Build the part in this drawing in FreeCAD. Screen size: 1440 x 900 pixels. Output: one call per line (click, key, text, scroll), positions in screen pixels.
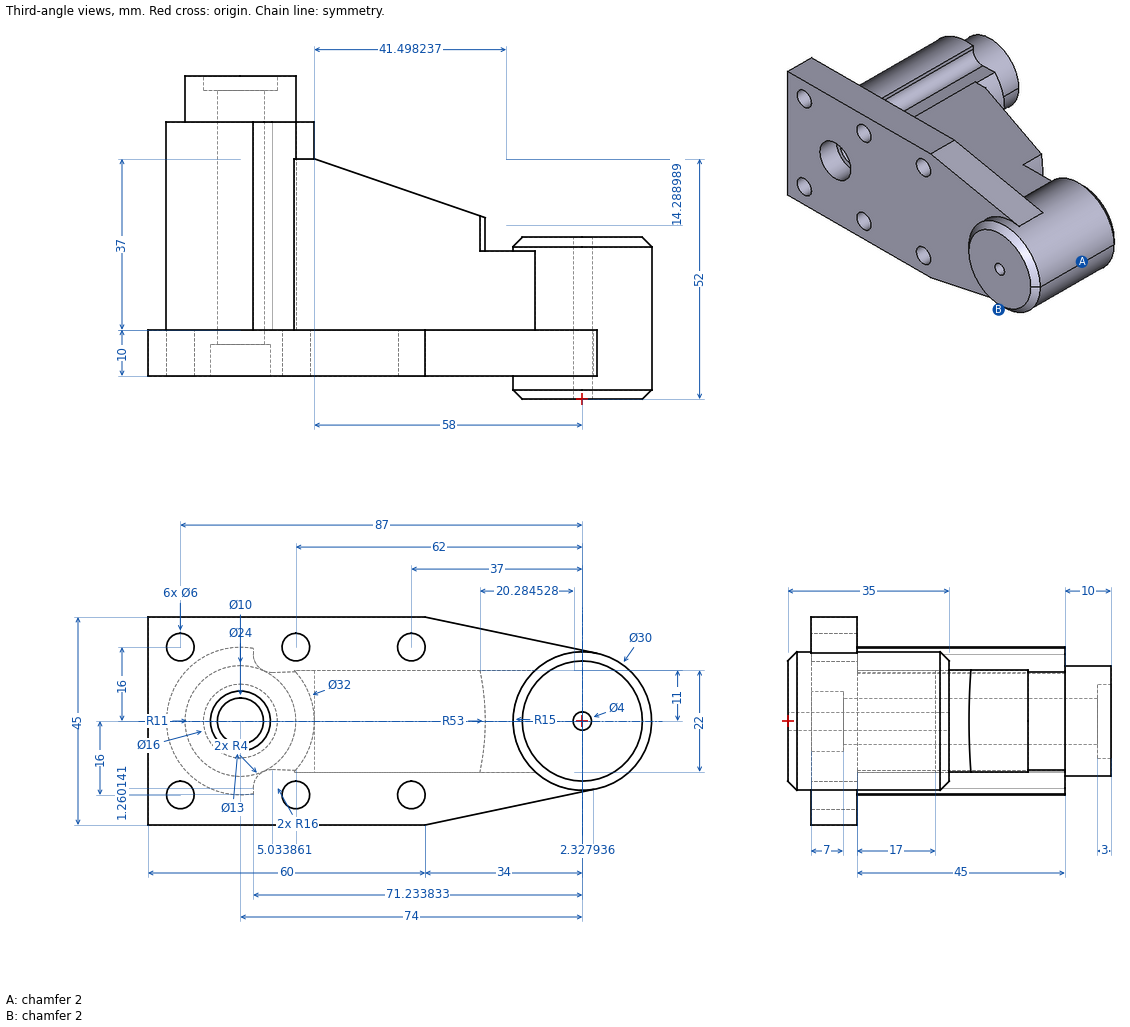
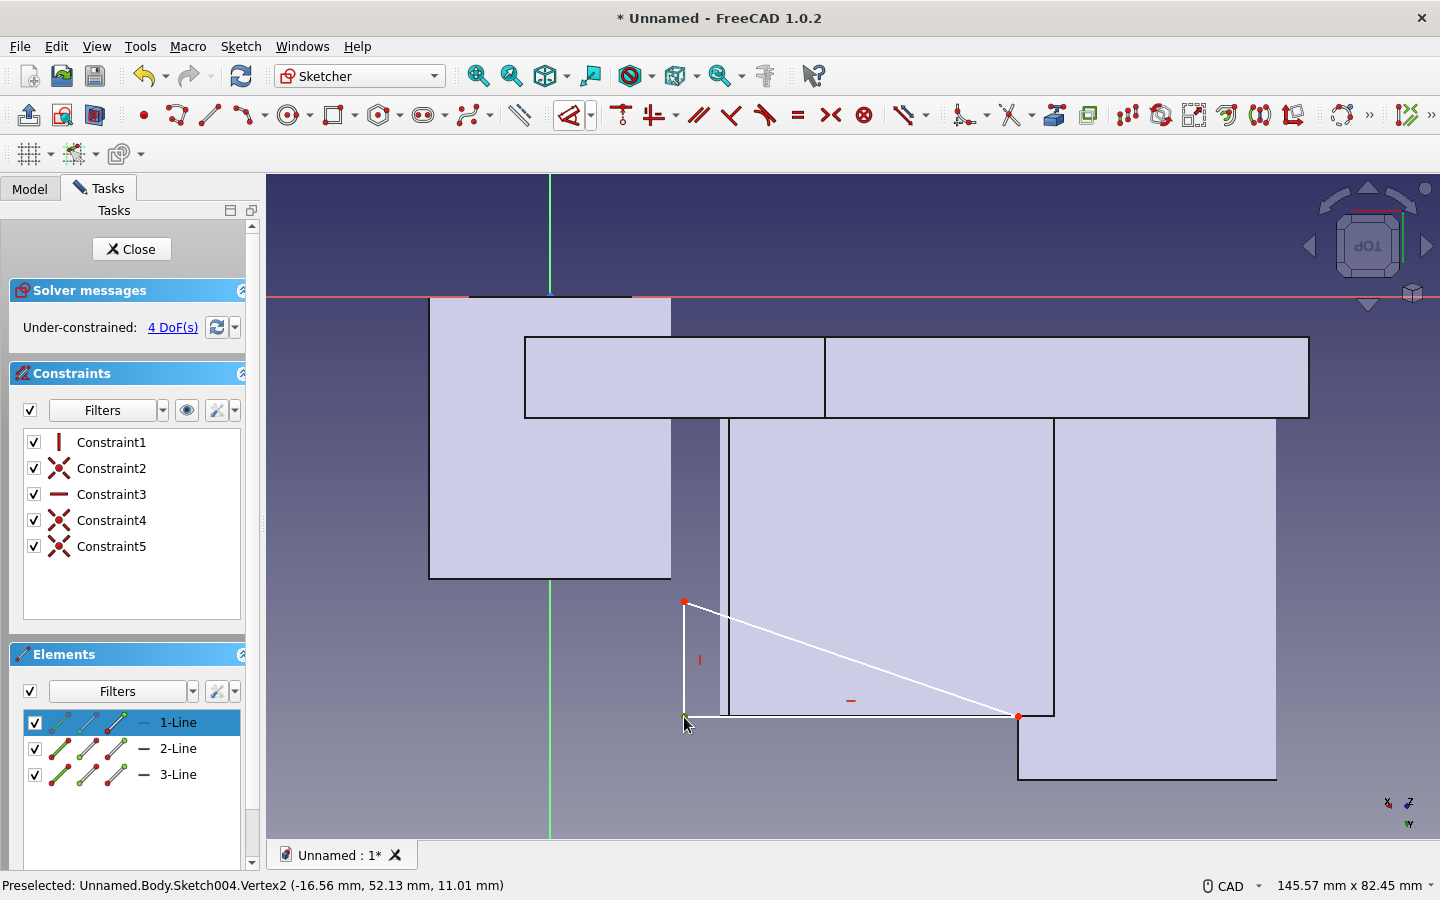
click(590, 116)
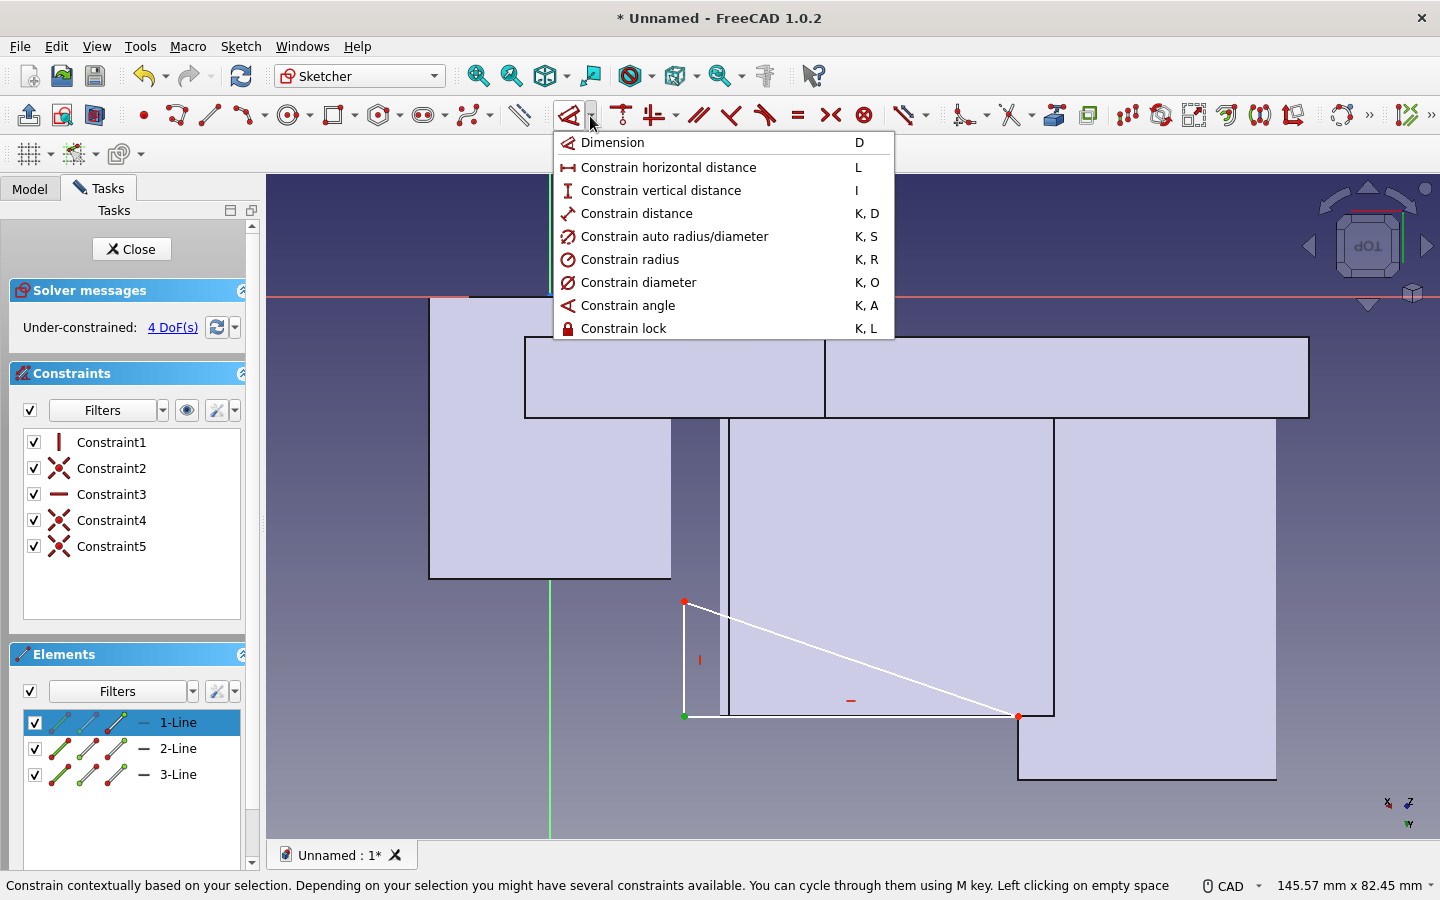
click(724, 190)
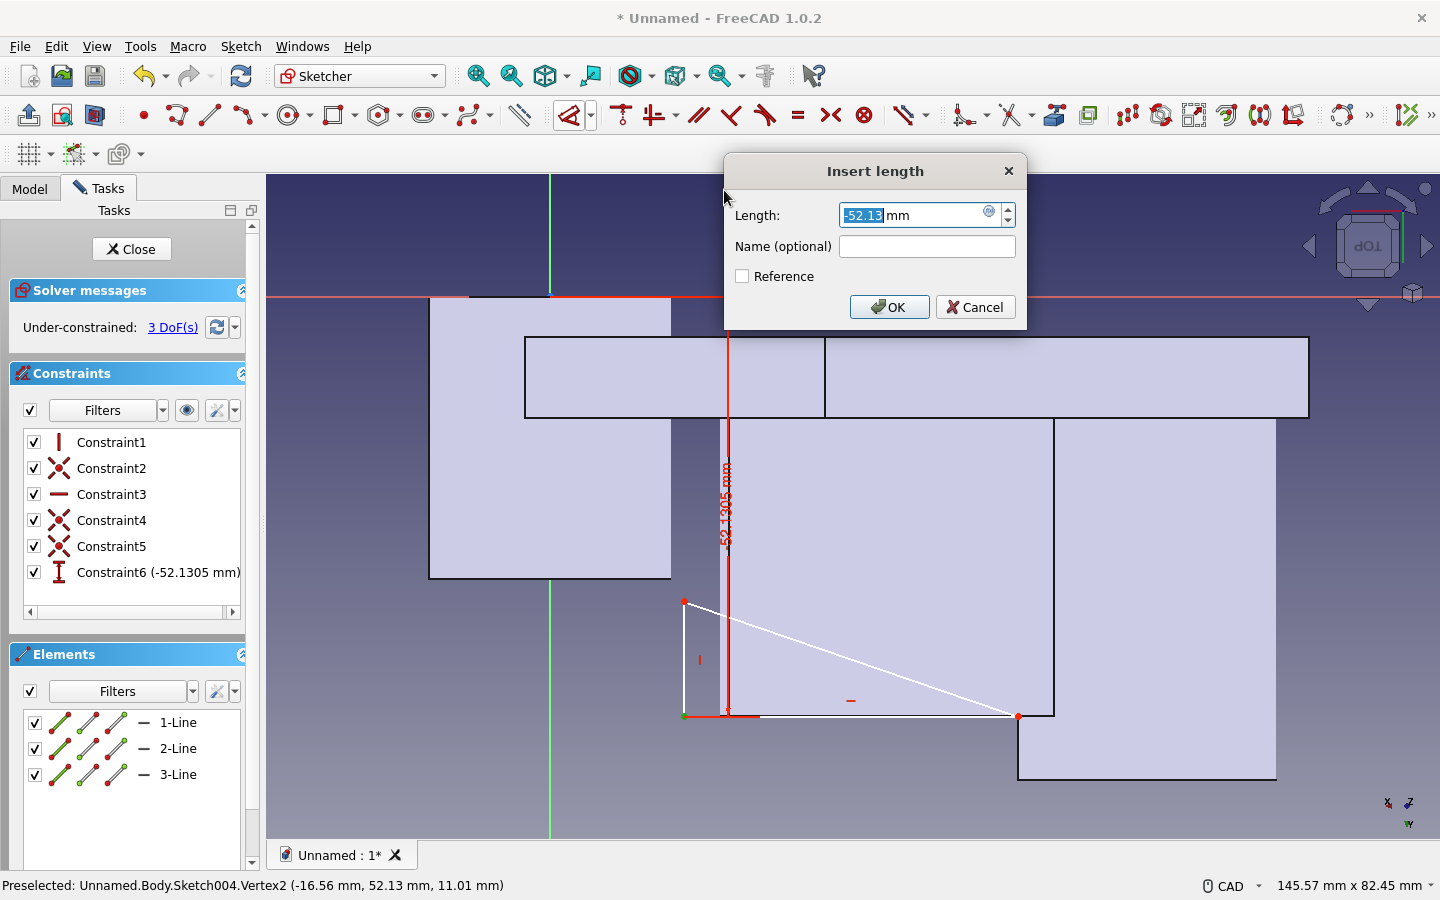
text(-52)
key(Return)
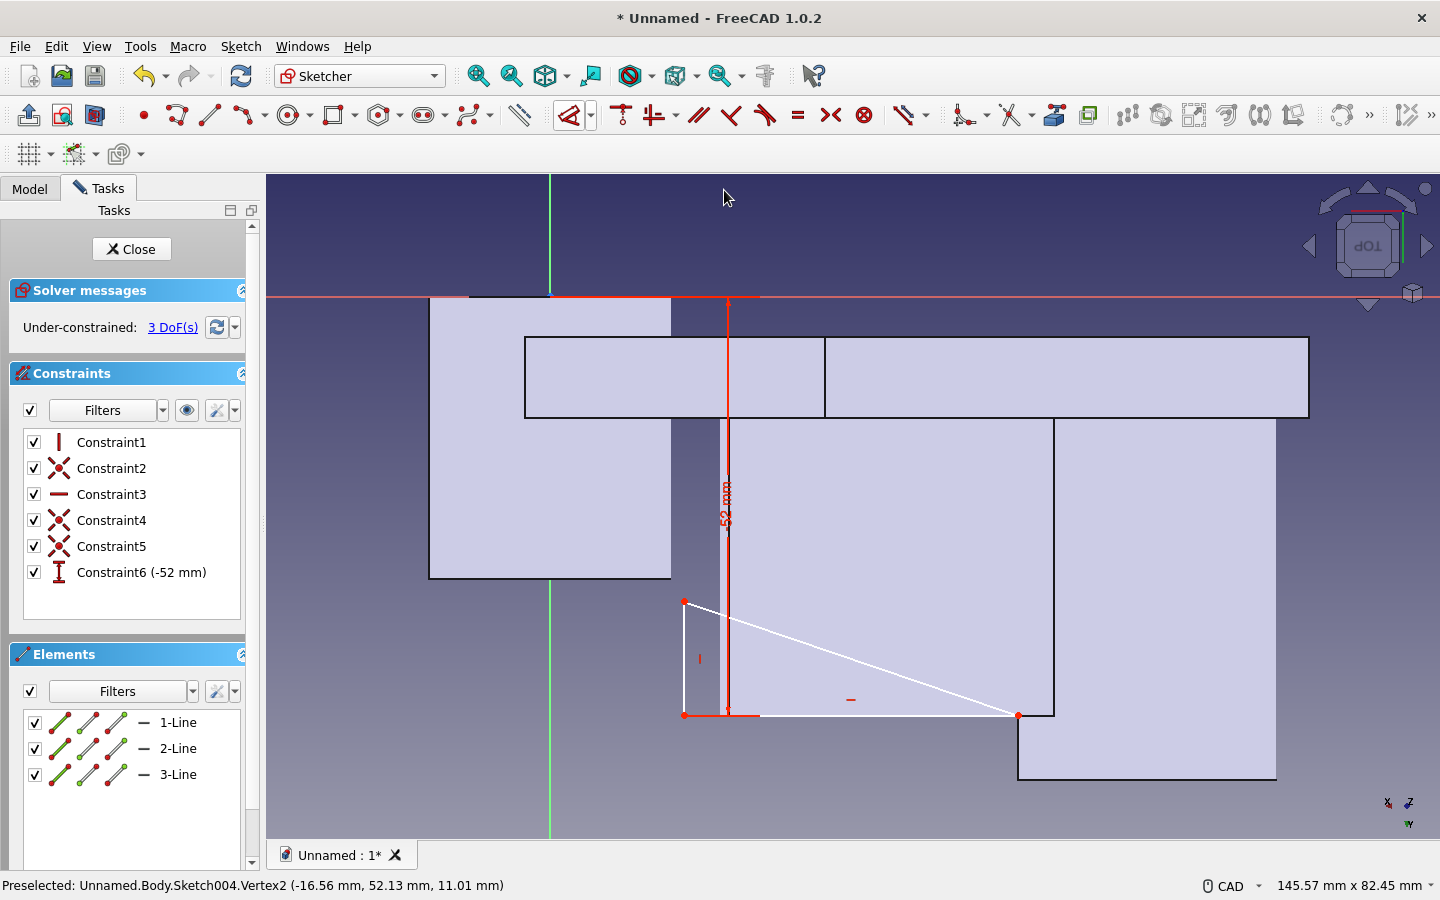
click(1018, 716)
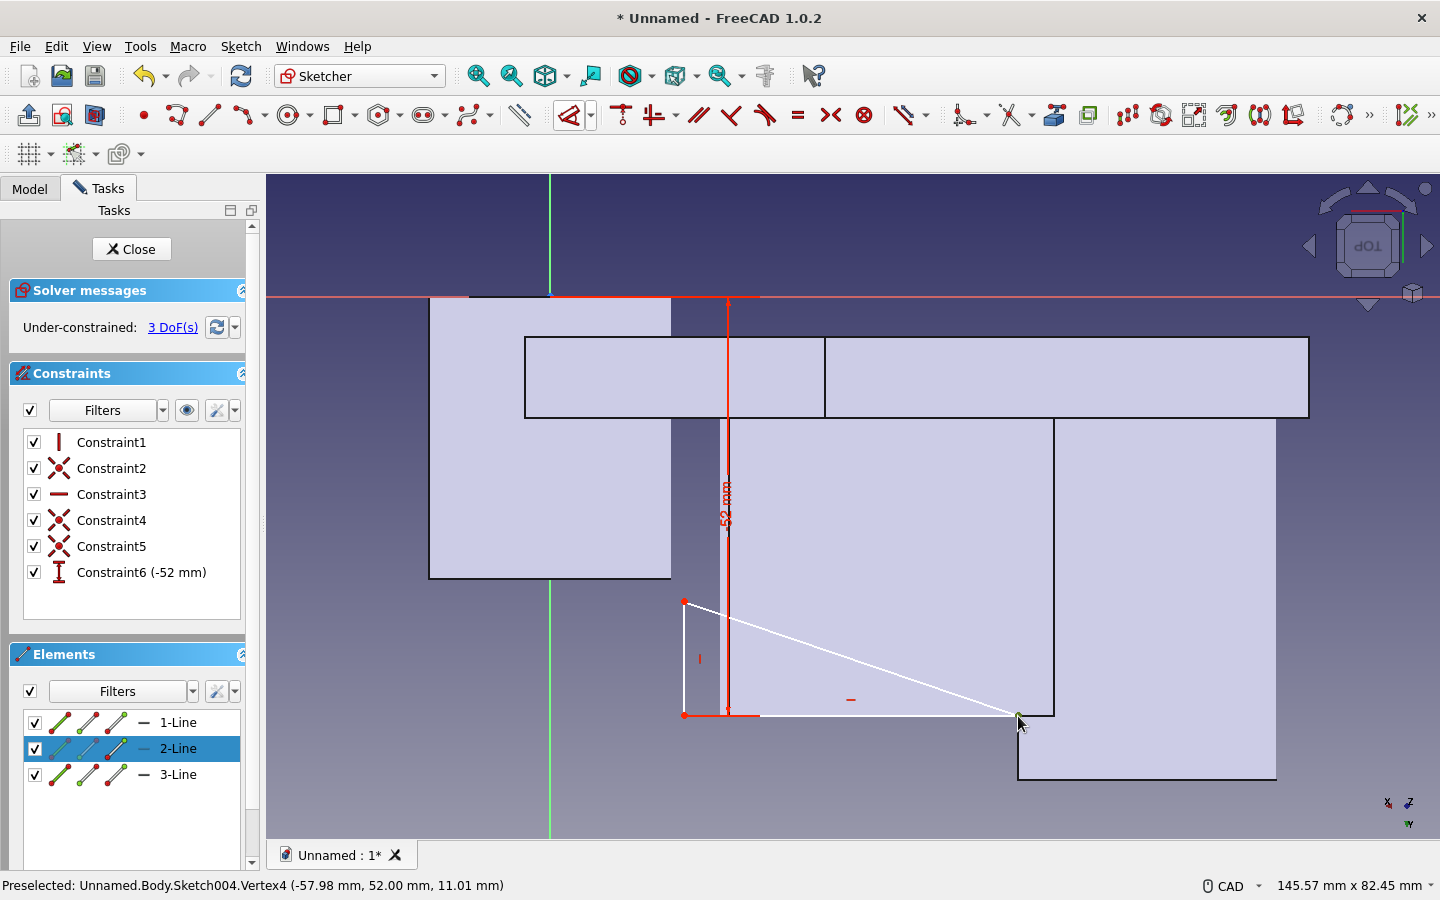
key(l)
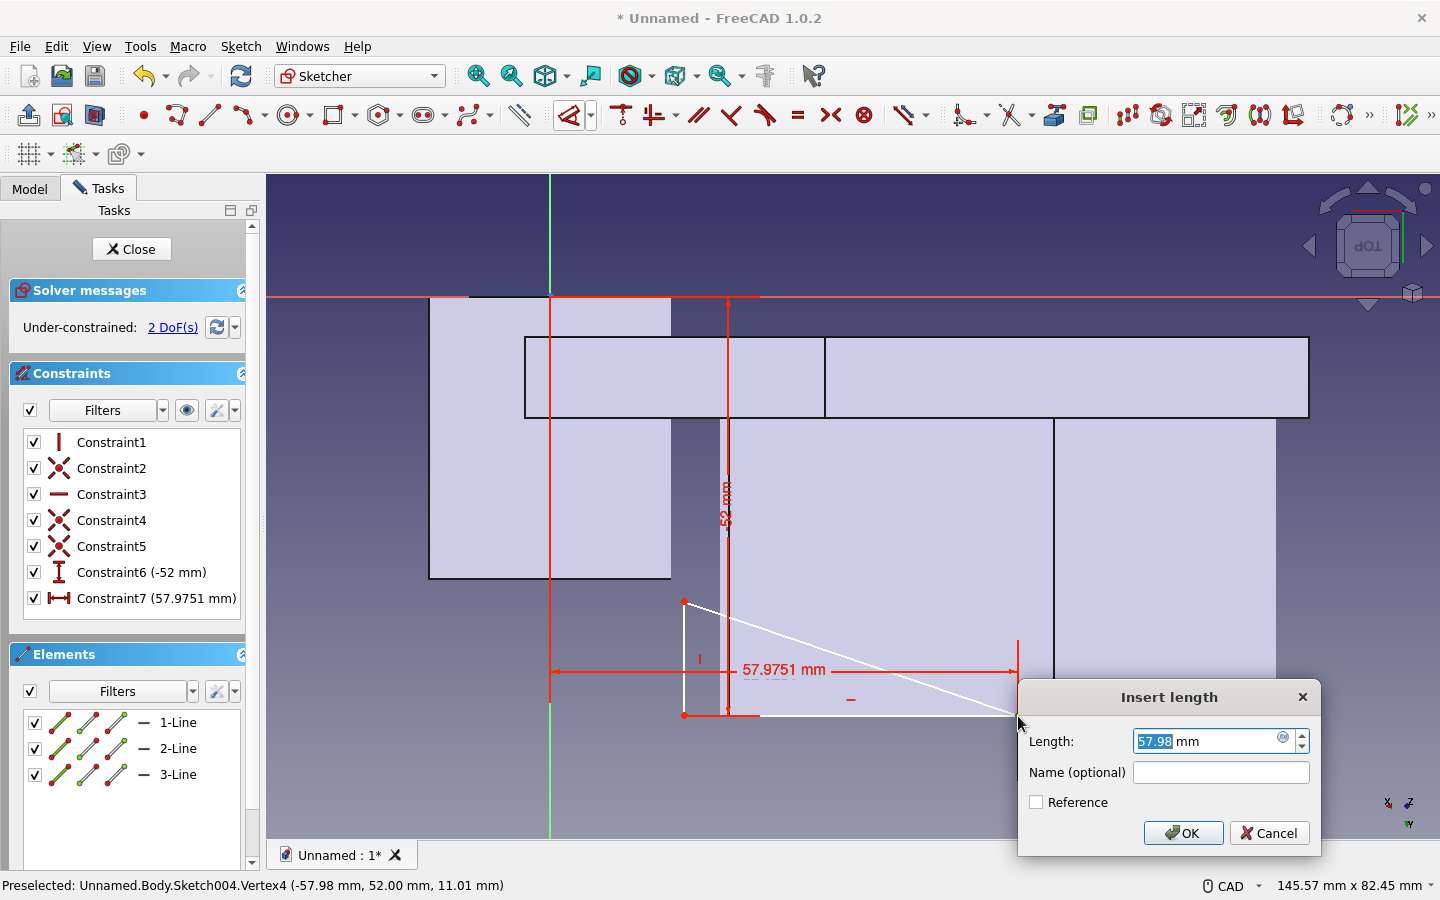
text(58)
key(Return)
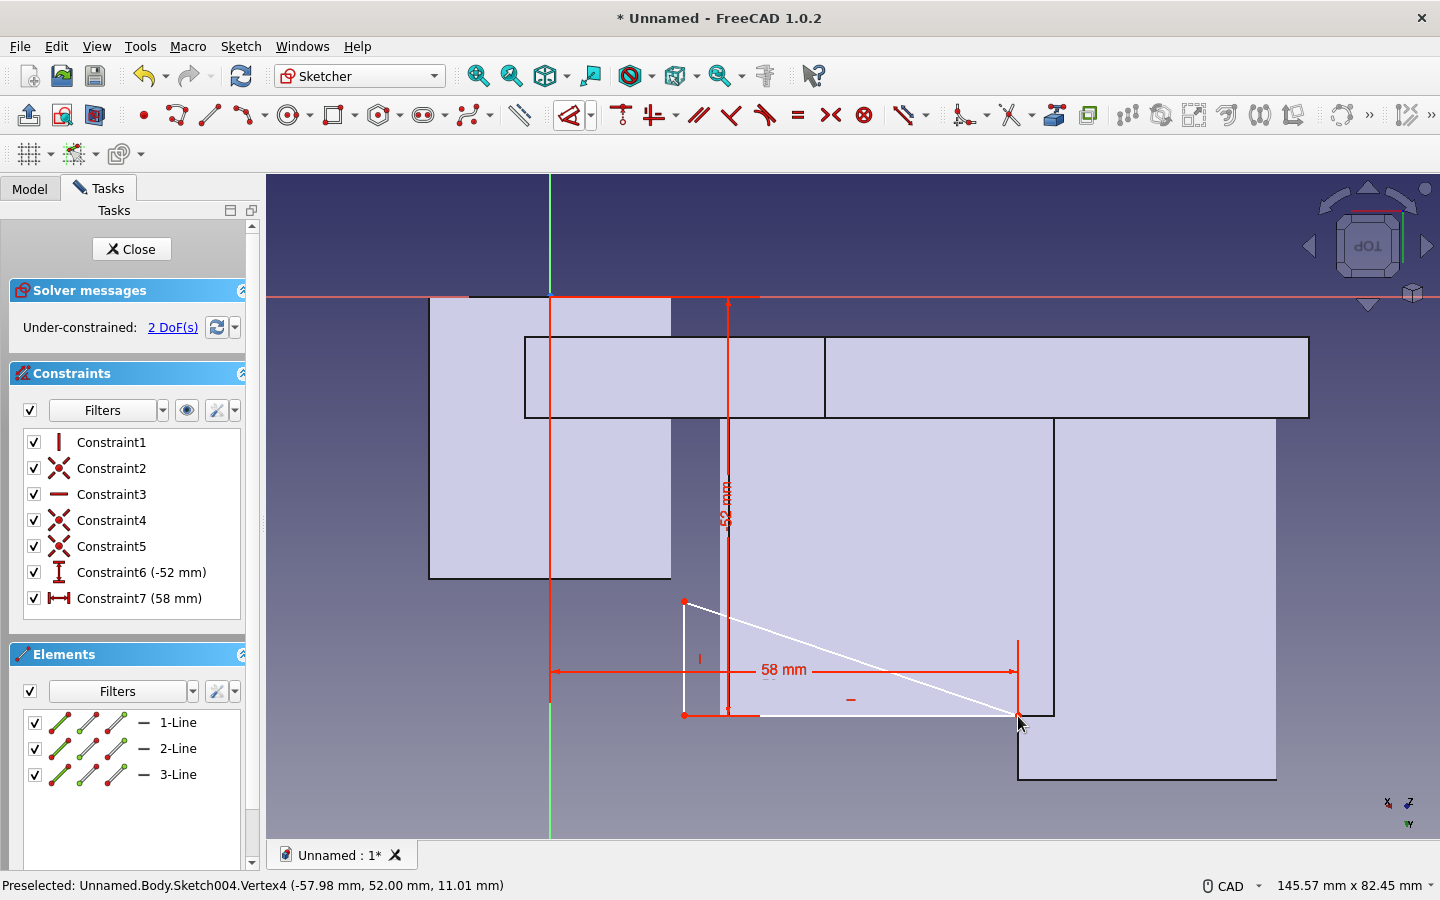
click(684, 636)